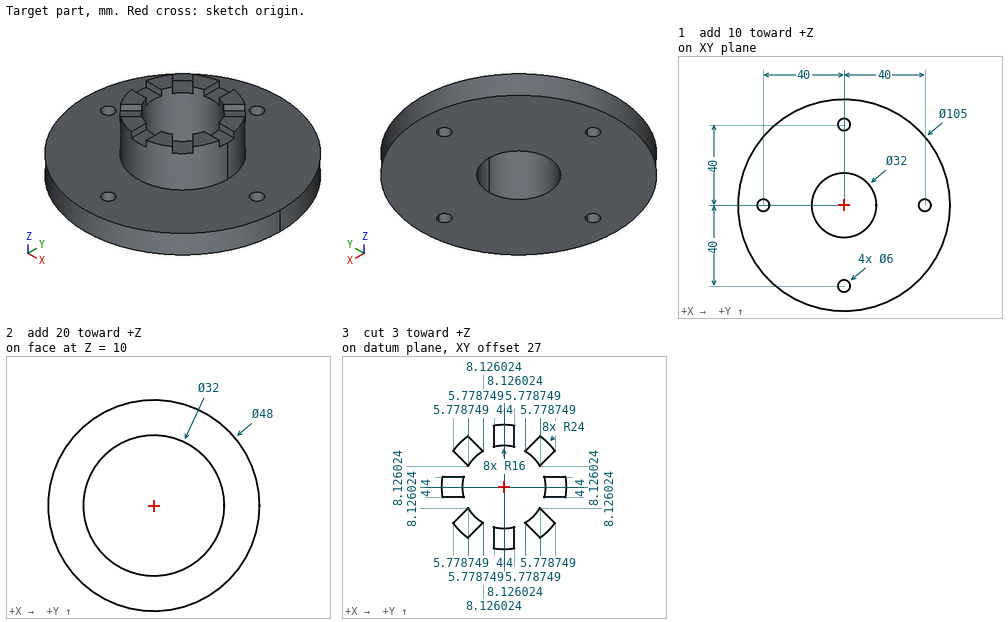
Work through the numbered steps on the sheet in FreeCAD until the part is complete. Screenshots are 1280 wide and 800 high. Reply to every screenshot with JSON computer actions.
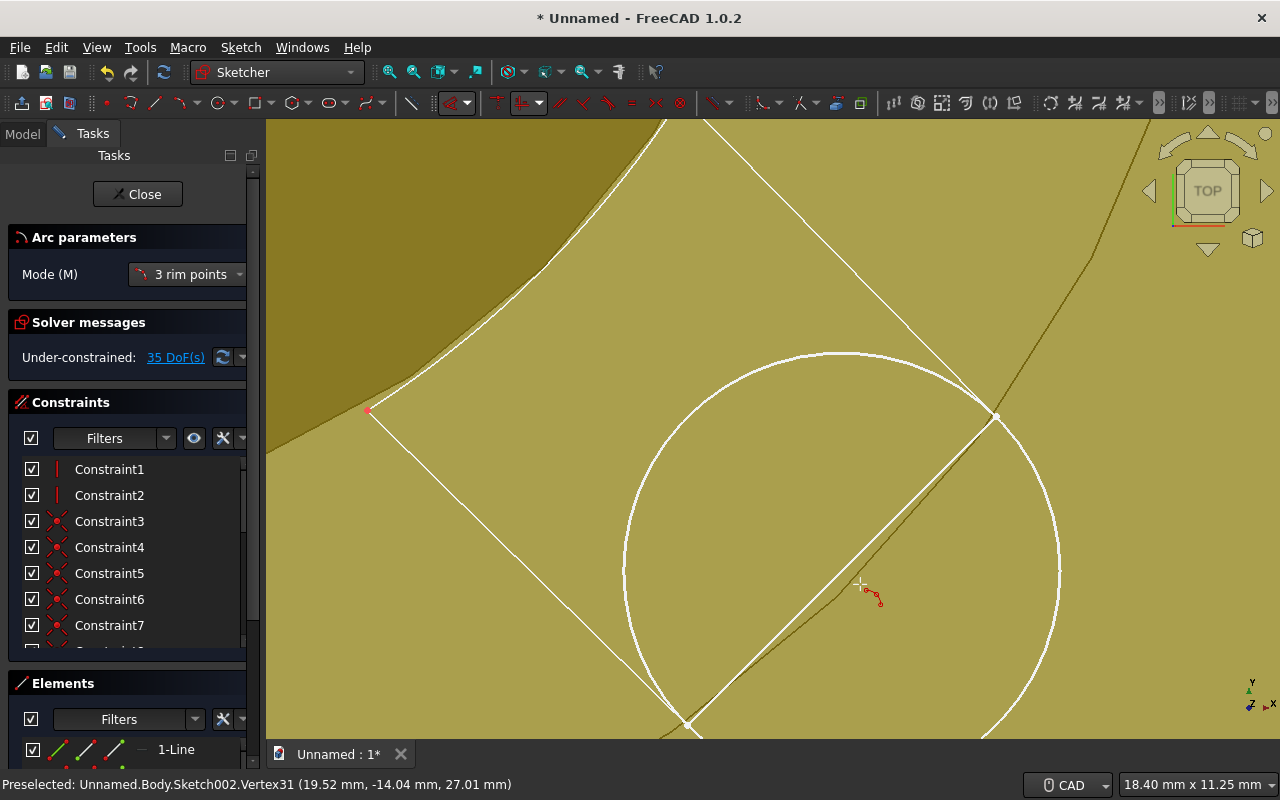
{"action": "left_click", "coordinate": [856, 578]}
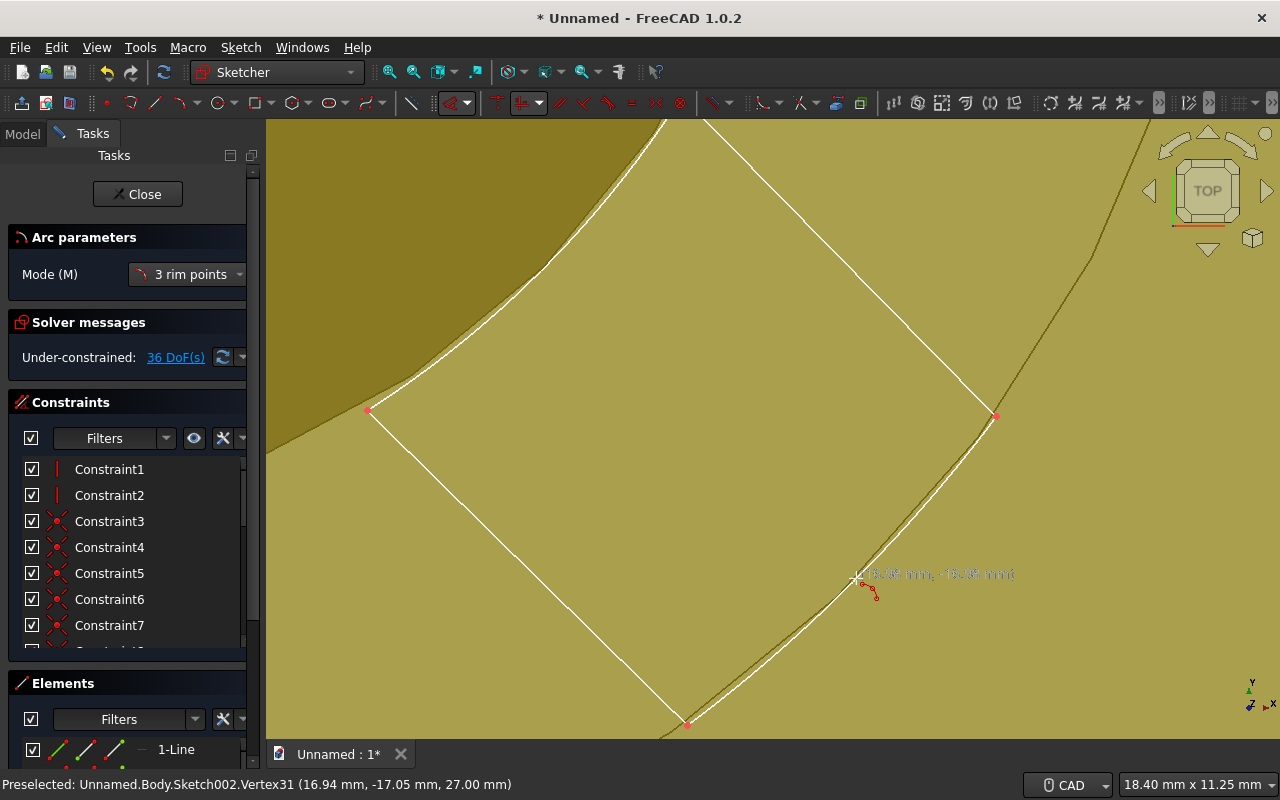
{"action": "left_click", "coordinate": [156, 104]}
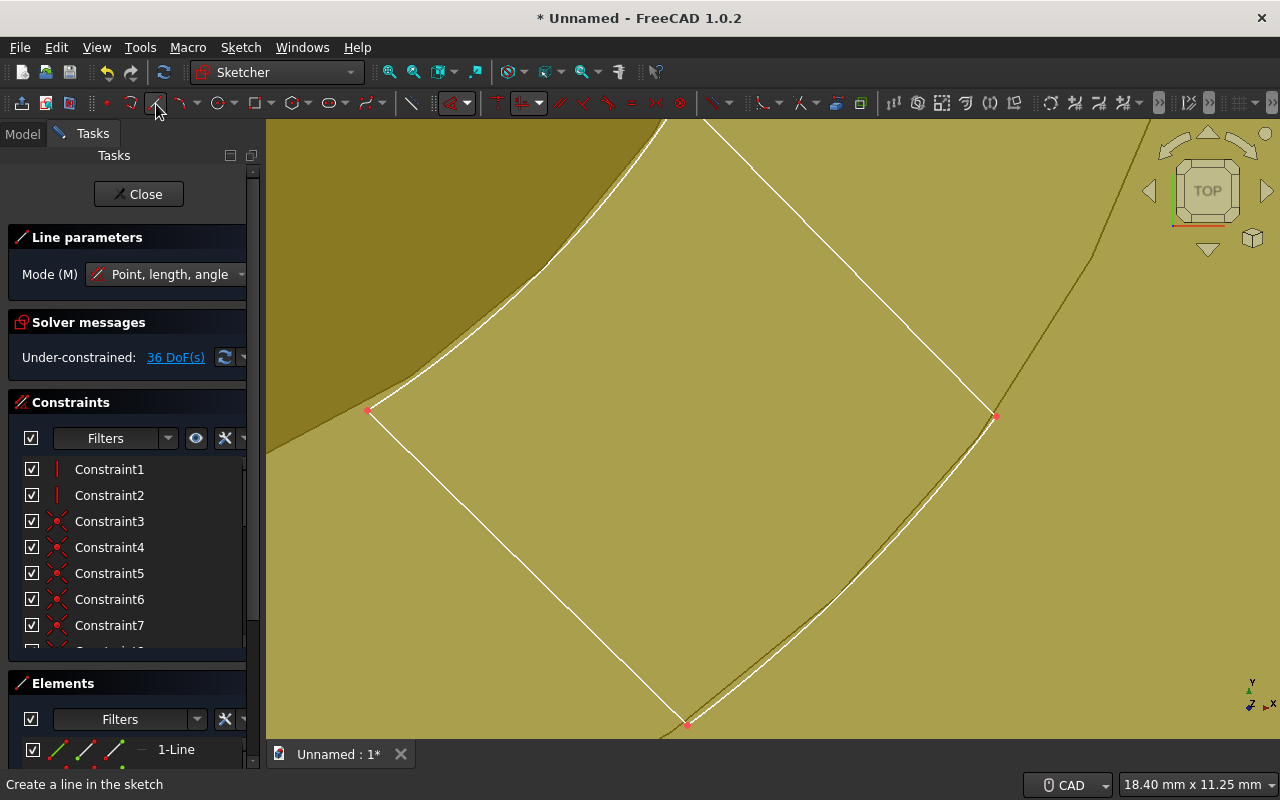
{"action": "scroll", "coordinate": [860, 585], "scroll_direction": "down", "scroll_amount": 9}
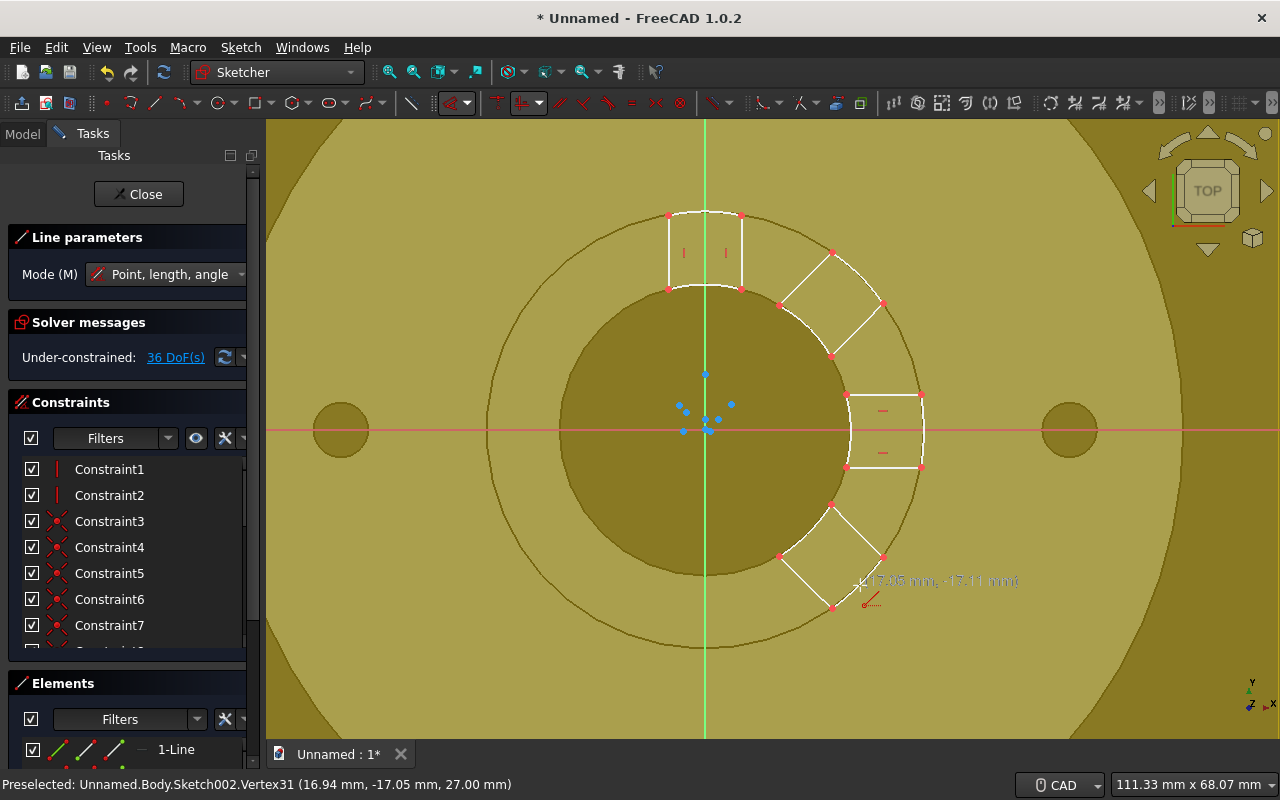
{"action": "left_click", "coordinate": [742, 646]}
{"action": "left_click", "coordinate": [742, 571]}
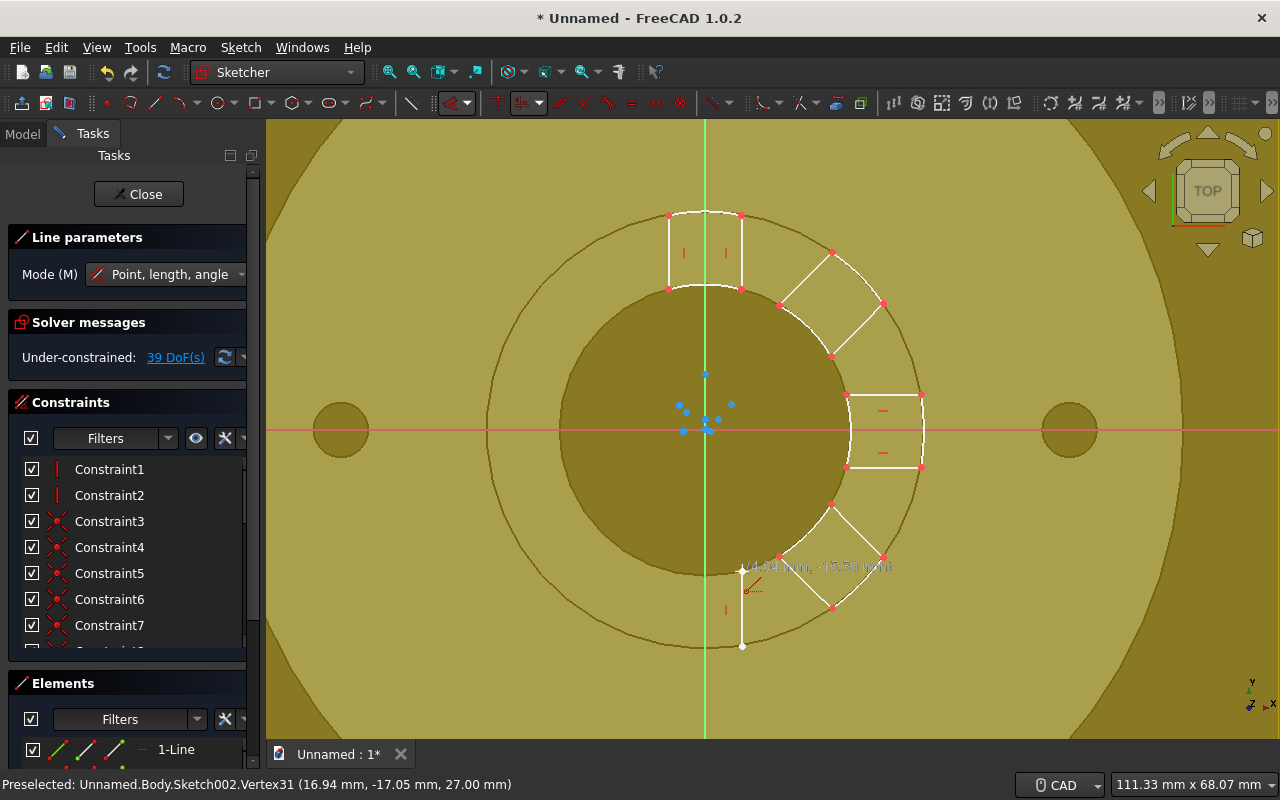
{"action": "left_click", "coordinate": [669, 571]}
{"action": "left_click", "coordinate": [669, 646]}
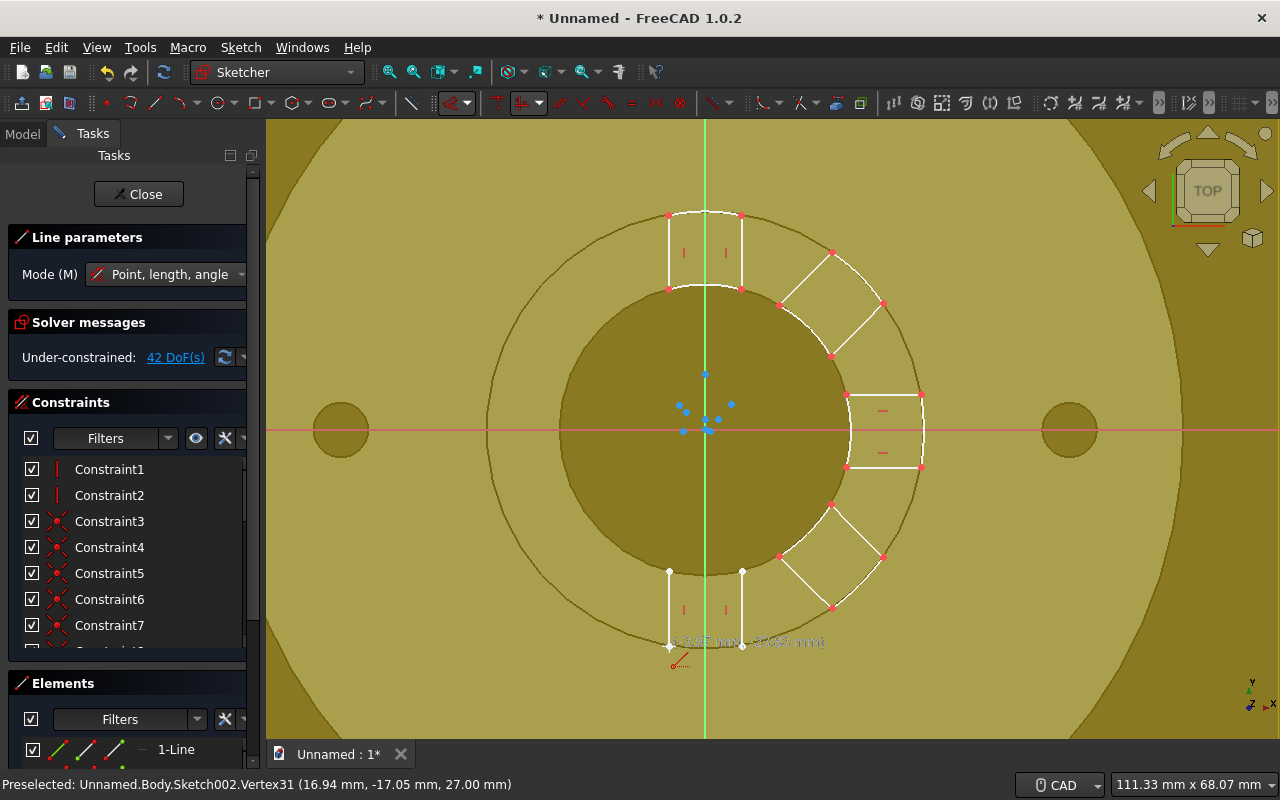
{"action": "left_click", "coordinate": [180, 104]}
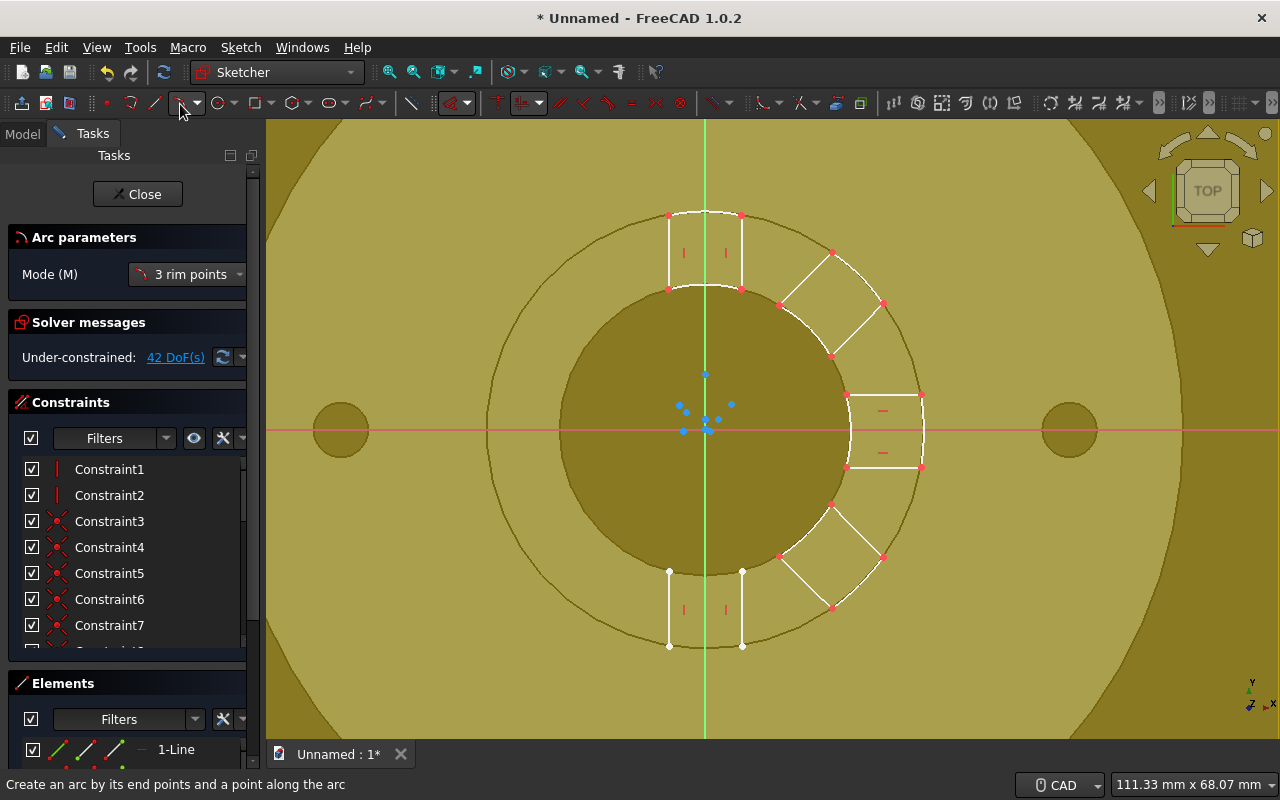
{"action": "left_click", "coordinate": [742, 572]}
{"action": "left_click", "coordinate": [669, 572]}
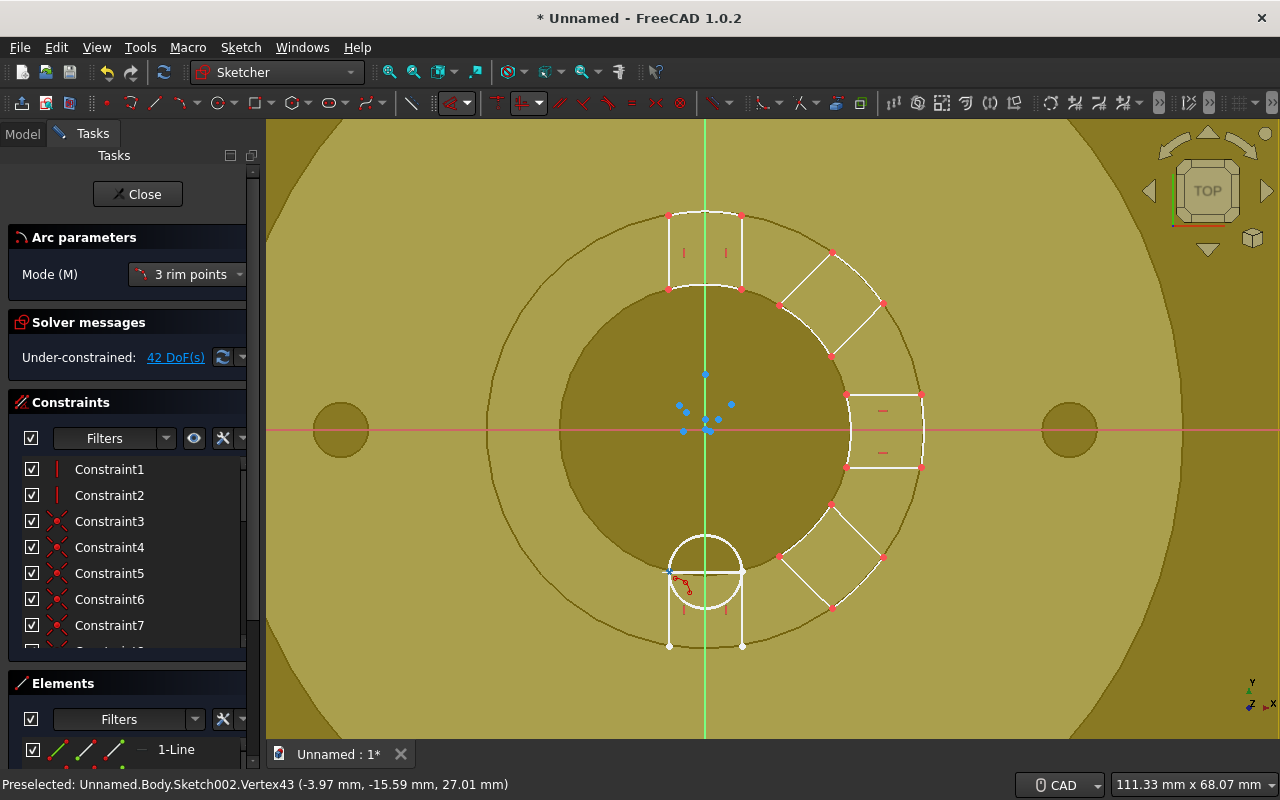
{"action": "scroll", "coordinate": [698, 576], "scroll_direction": "up", "scroll_amount": 7}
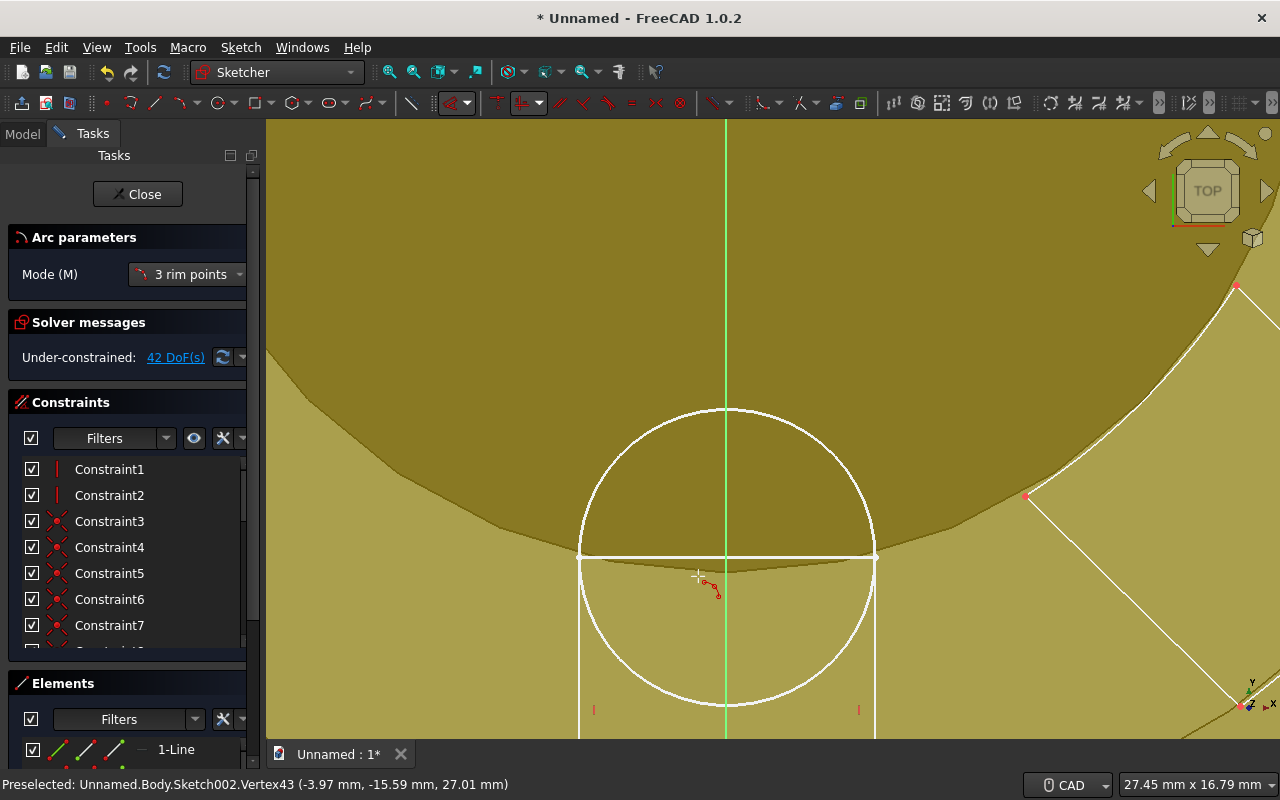
{"action": "left_click", "coordinate": [696, 572]}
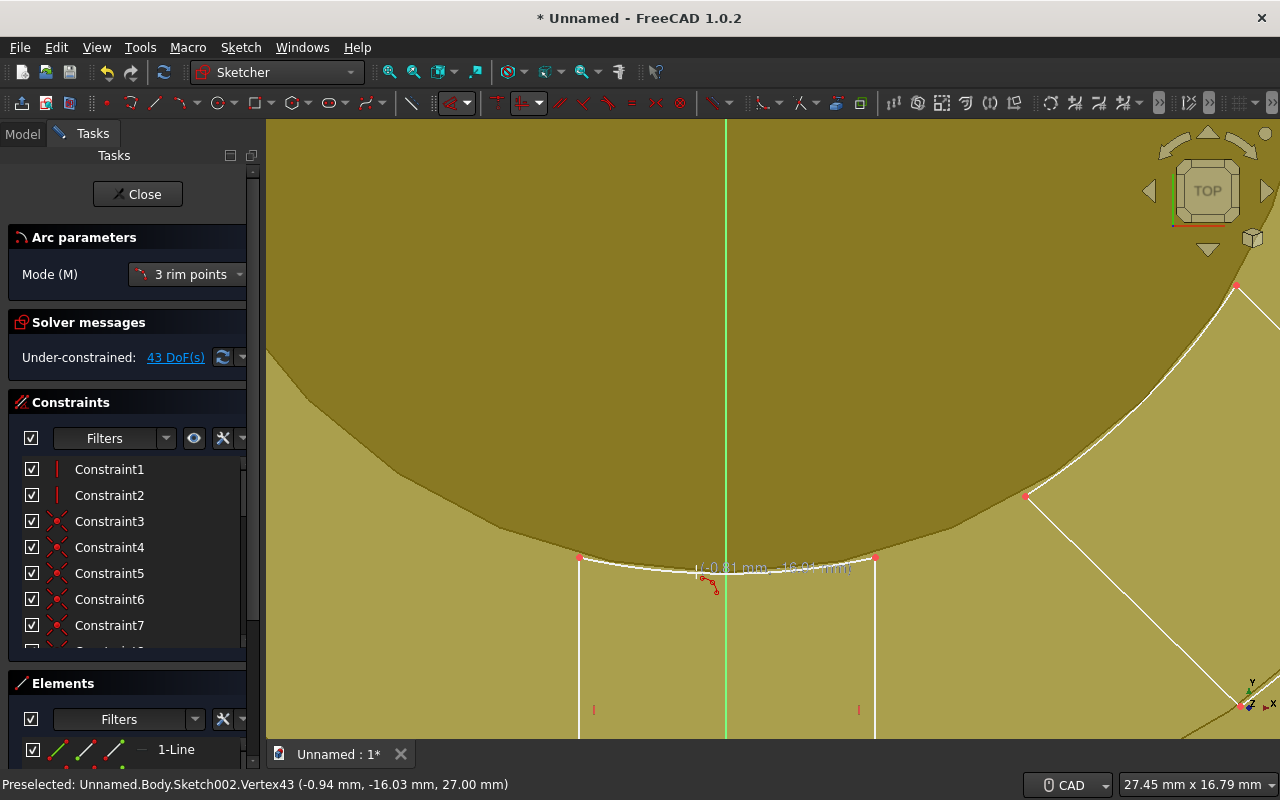
{"action": "scroll", "coordinate": [698, 575], "scroll_direction": "down", "scroll_amount": 7}